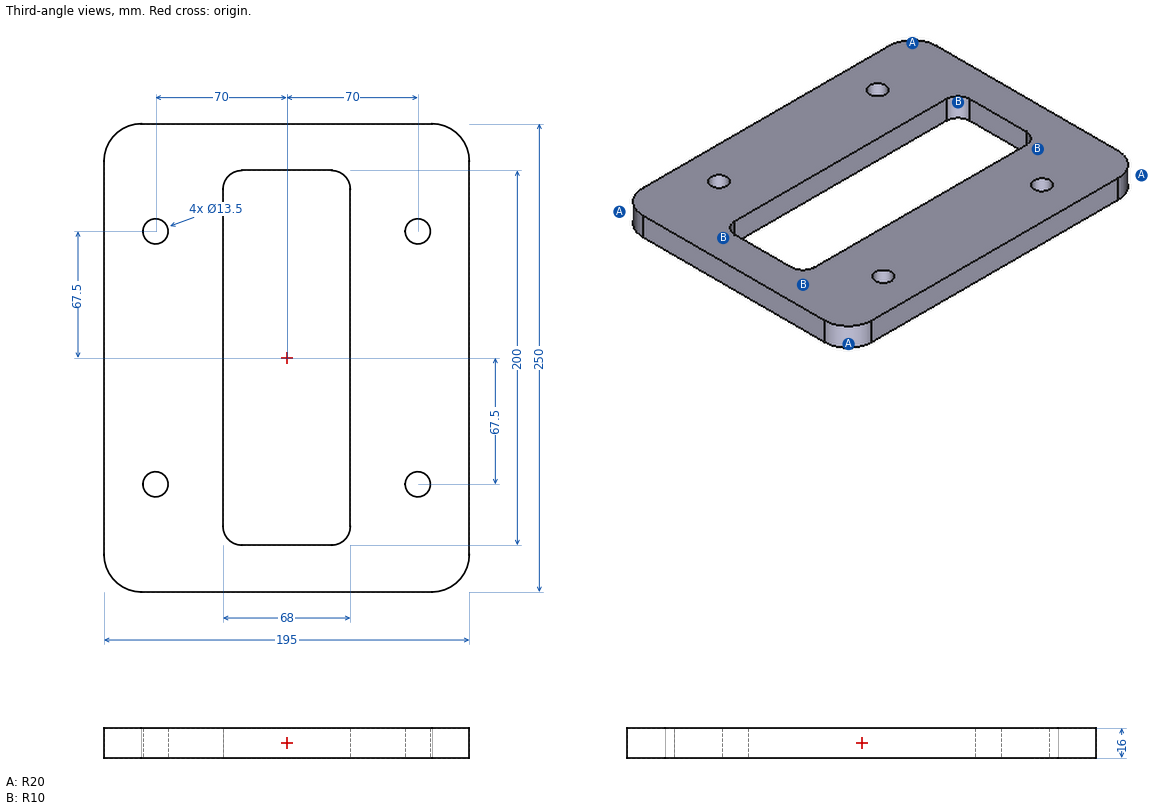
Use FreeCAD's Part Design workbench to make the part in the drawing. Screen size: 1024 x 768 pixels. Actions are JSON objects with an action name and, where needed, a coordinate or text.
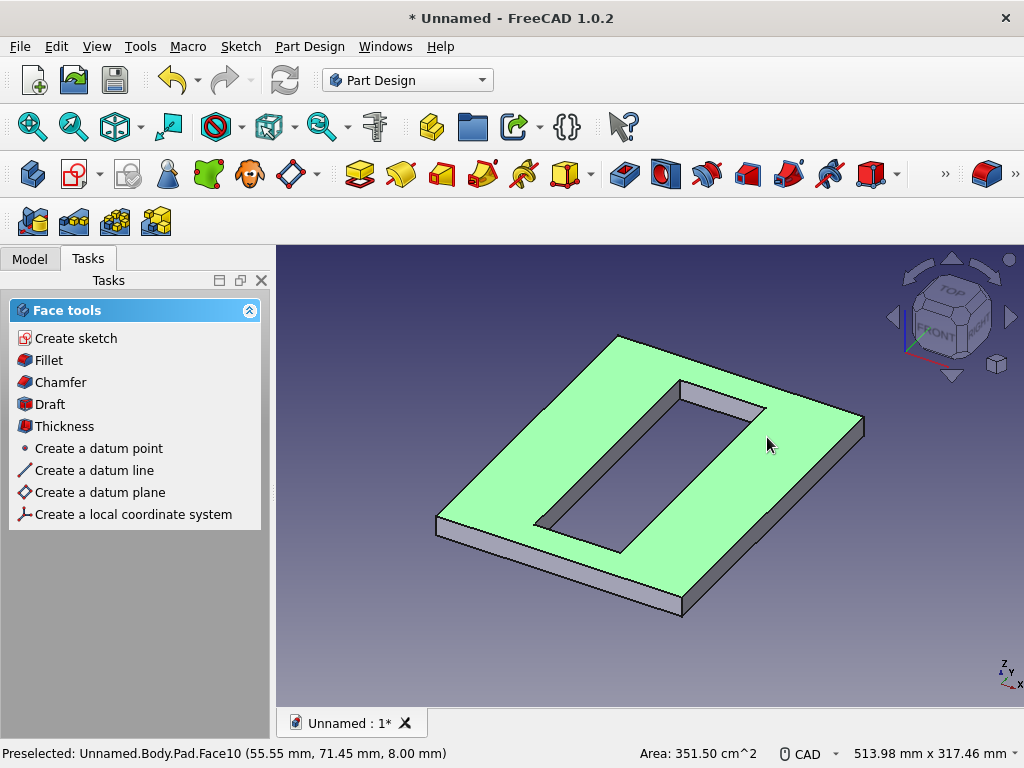
{"action": "left_click", "coordinate": [74, 174]}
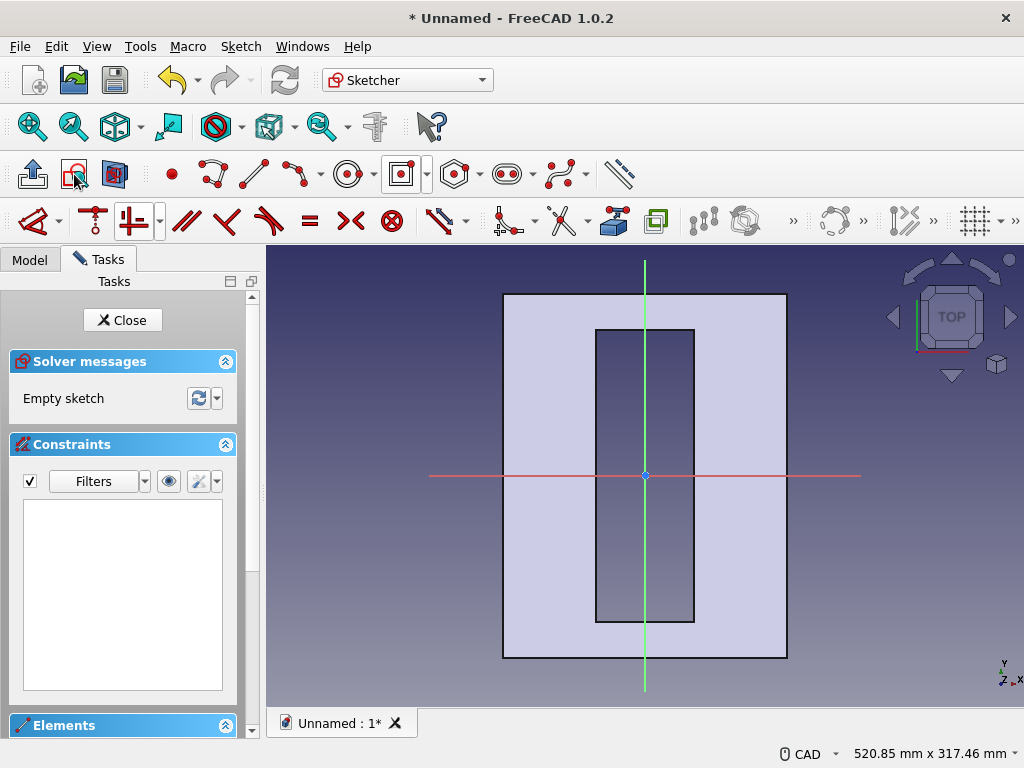
{"action": "left_click", "coordinate": [348, 174]}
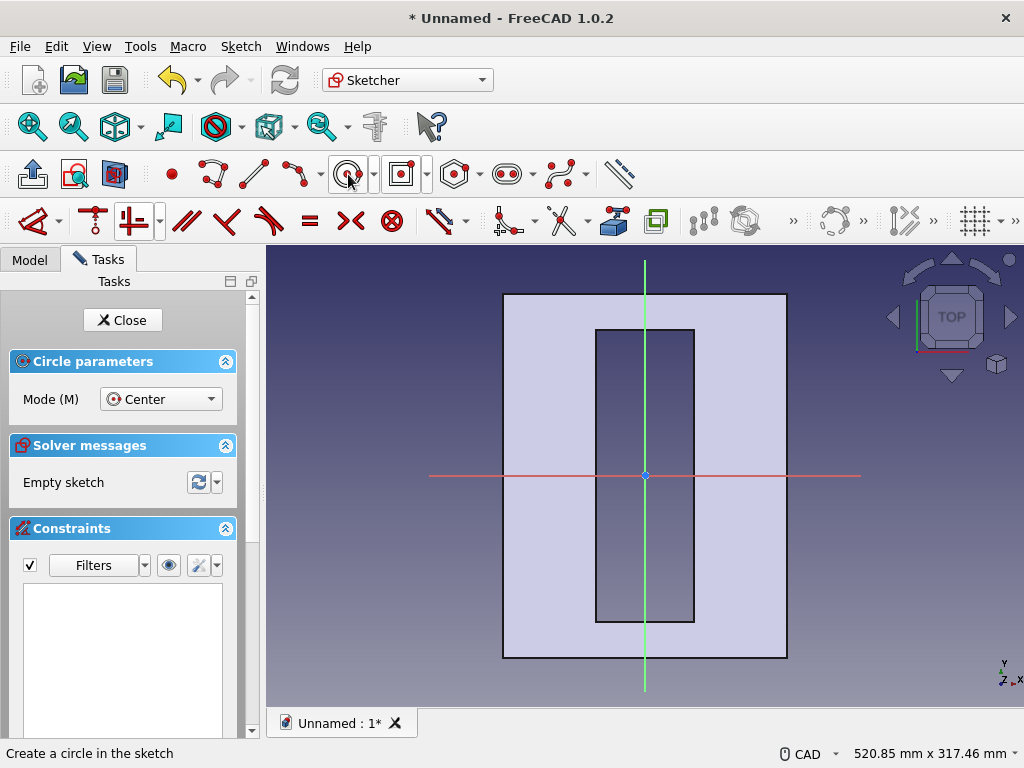
{"action": "scroll", "coordinate": [543, 378], "scroll_direction": "up", "scroll_amount": 5}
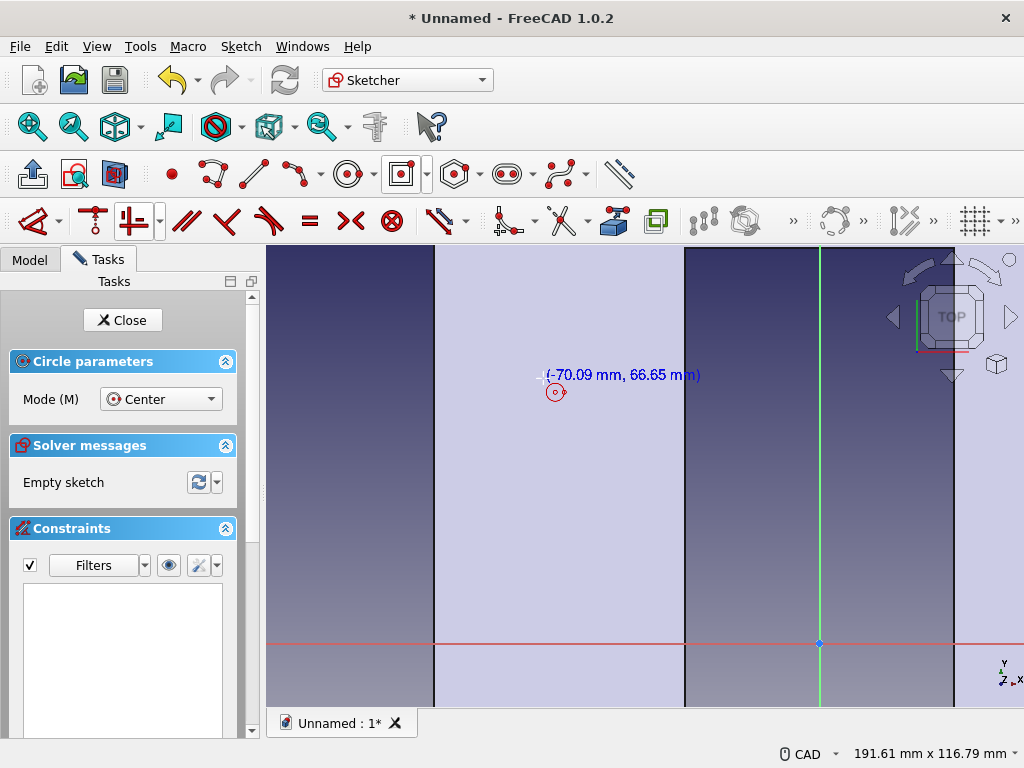
{"action": "left_click", "coordinate": [543, 377]}
{"action": "left_click", "coordinate": [562, 358]}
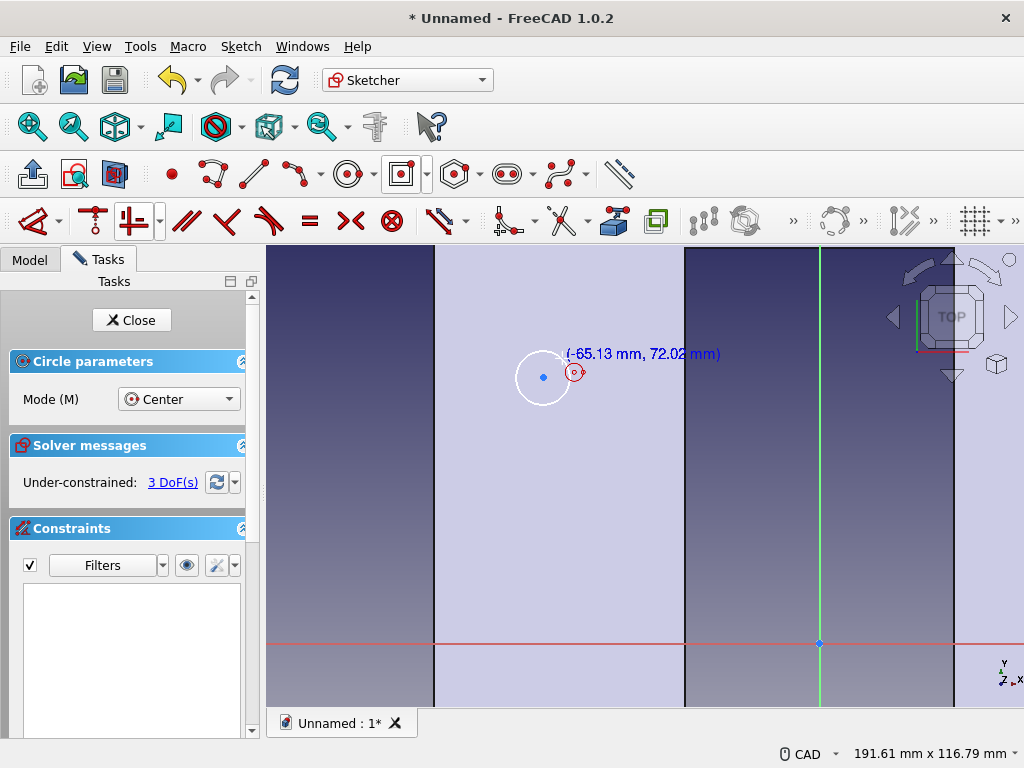
{"action": "scroll", "coordinate": [378, 339], "scroll_direction": "down", "scroll_amount": 4}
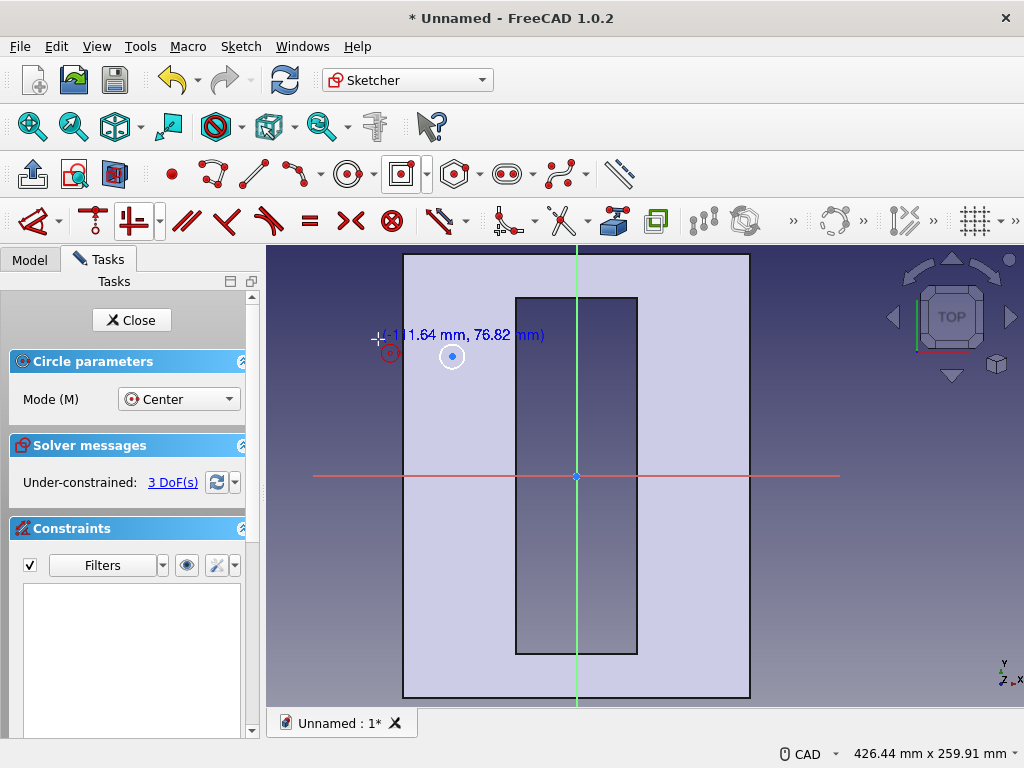
{"action": "scroll", "coordinate": [701, 356], "scroll_direction": "up", "scroll_amount": 4}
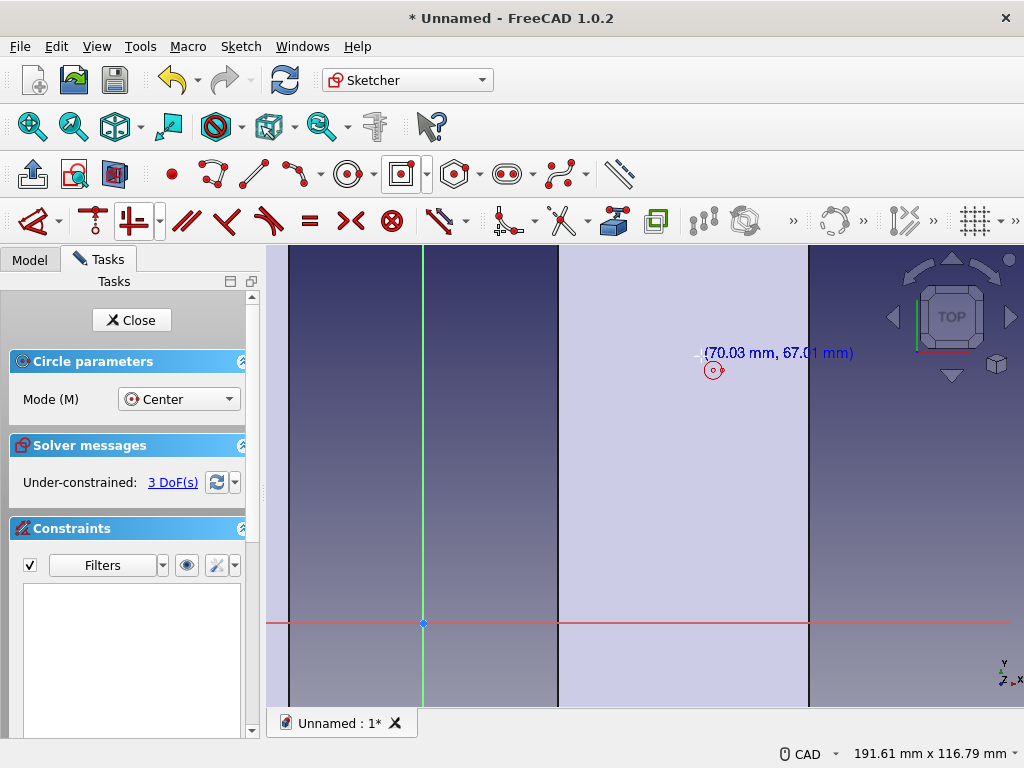
{"action": "left_click", "coordinate": [700, 356]}
{"action": "left_click", "coordinate": [719, 337]}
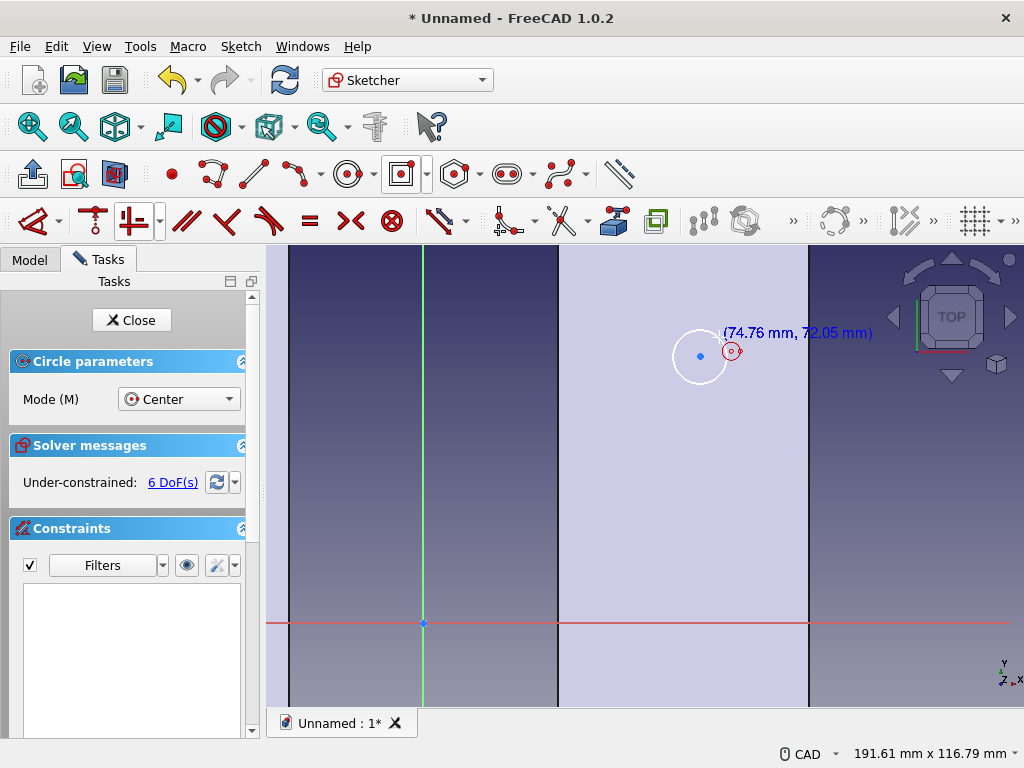
{"action": "scroll", "coordinate": [702, 356], "scroll_direction": "down", "scroll_amount": 4}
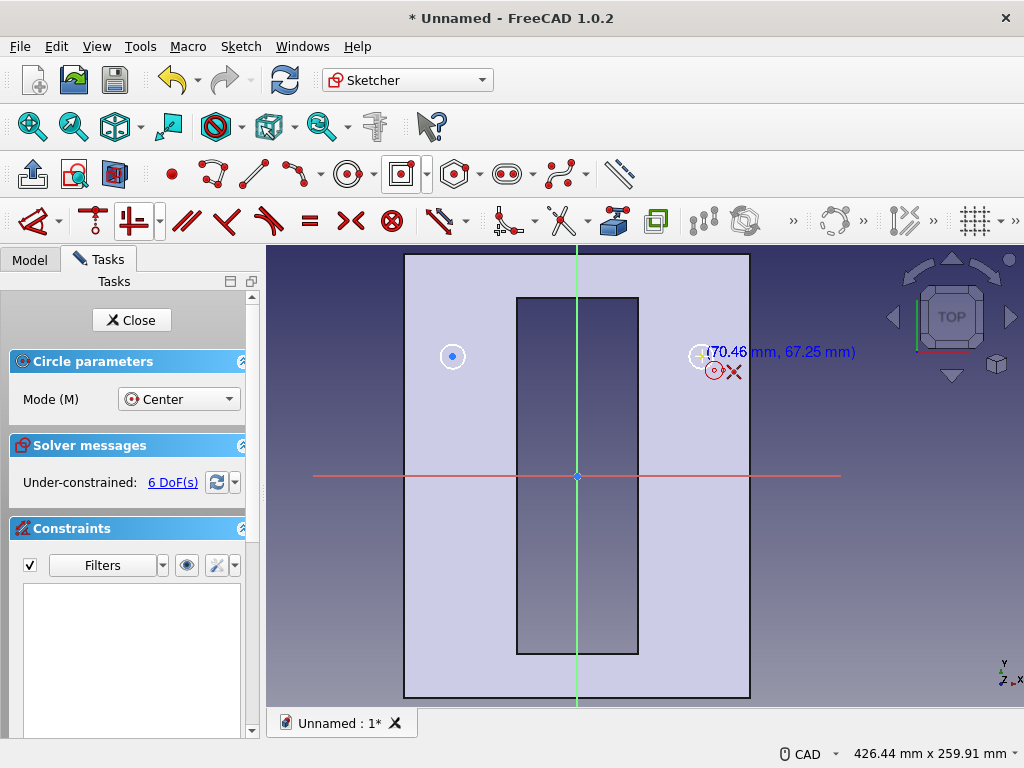
{"action": "scroll", "coordinate": [701, 596], "scroll_direction": "up", "scroll_amount": 4}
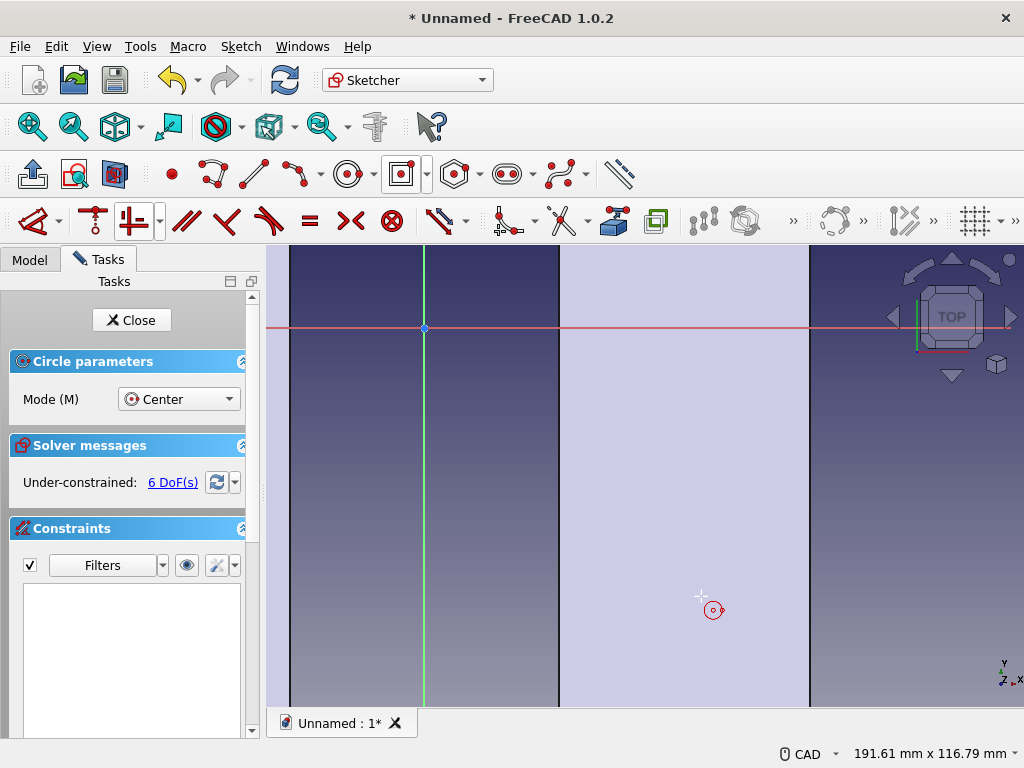
{"action": "left_click", "coordinate": [701, 595]}
{"action": "left_click", "coordinate": [720, 576]}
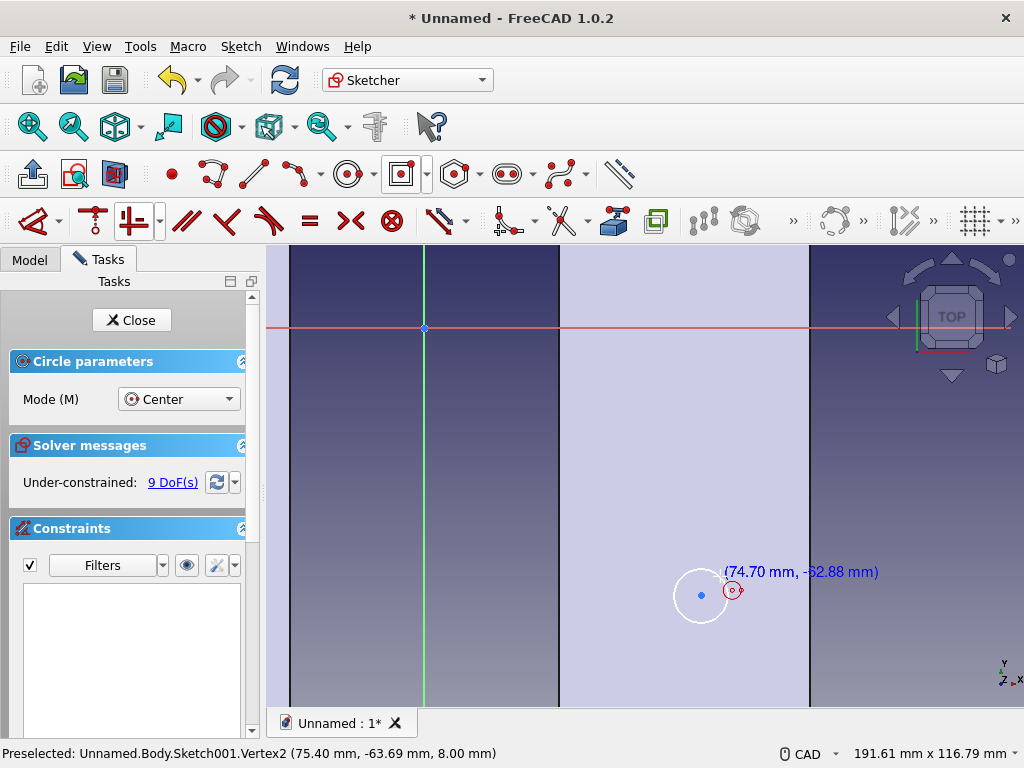
{"action": "scroll", "coordinate": [701, 597], "scroll_direction": "down", "scroll_amount": 4}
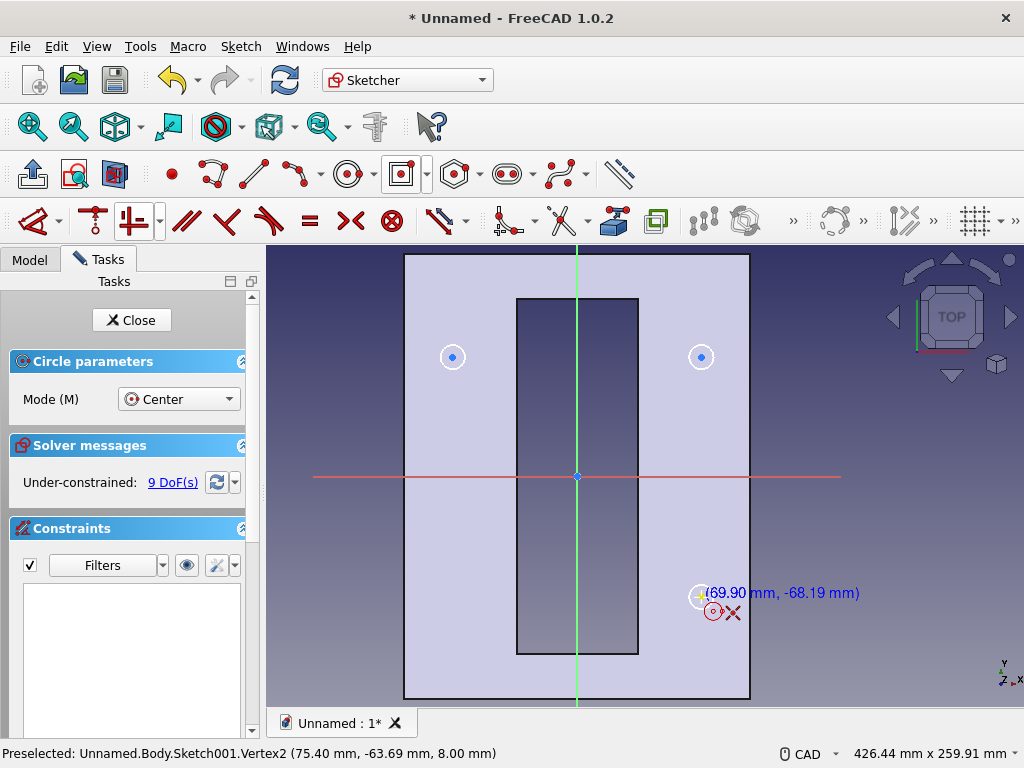
{"action": "scroll", "coordinate": [453, 597], "scroll_direction": "up", "scroll_amount": 4}